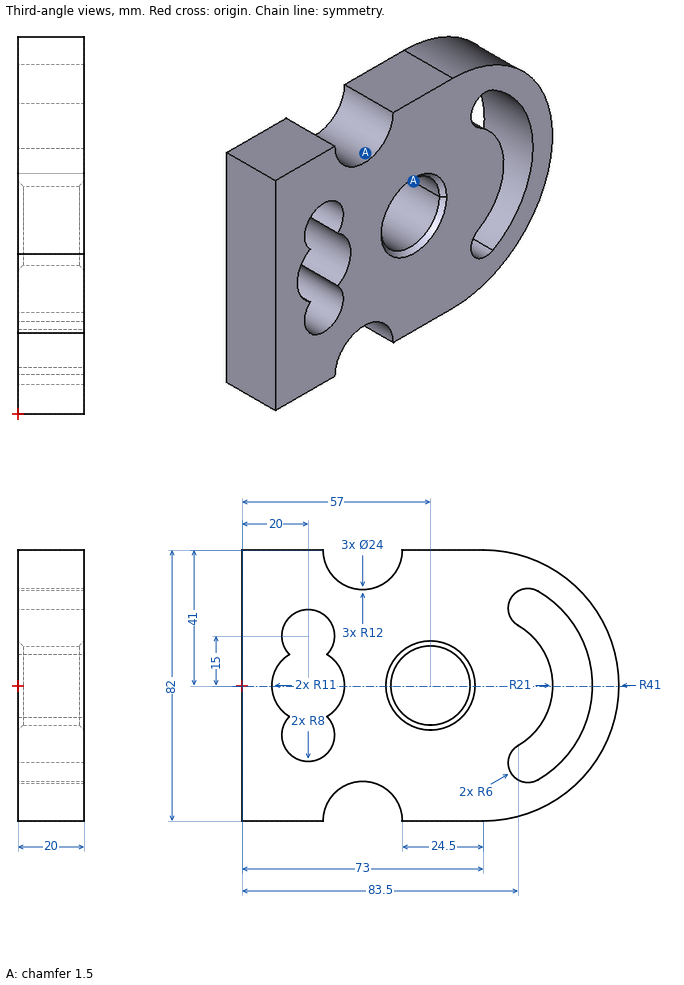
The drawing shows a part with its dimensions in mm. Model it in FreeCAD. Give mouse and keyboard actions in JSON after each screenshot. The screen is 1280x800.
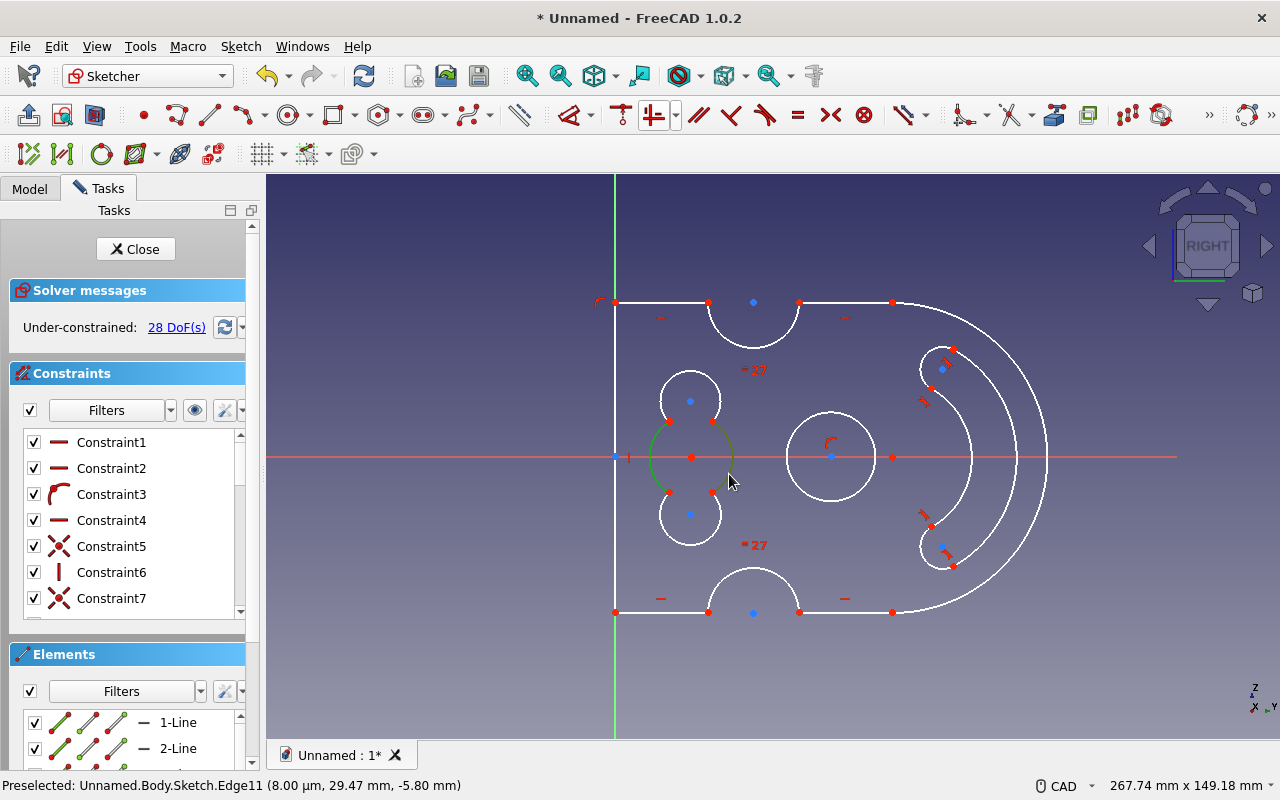
{"action": "key", "text": "e"}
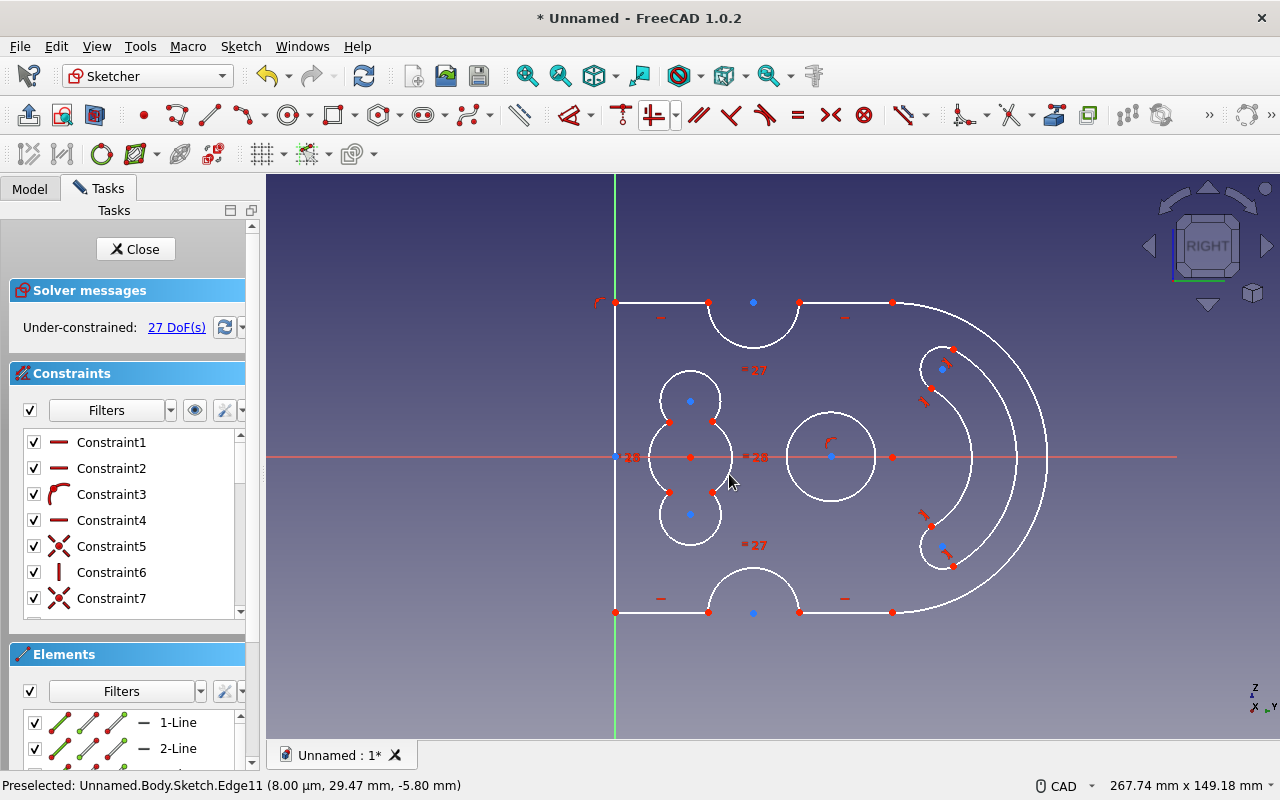
{"action": "left_click", "coordinate": [715, 383]}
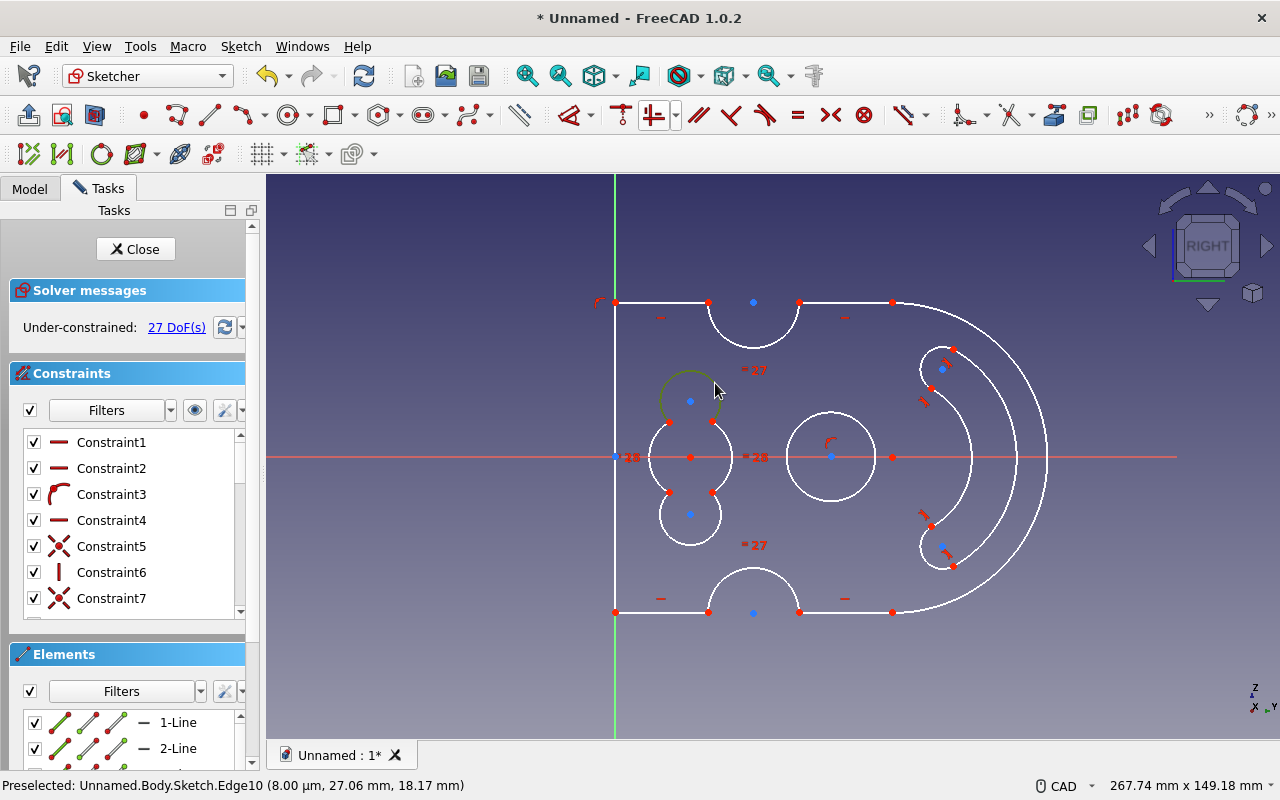
{"action": "left_click", "coordinate": [666, 532]}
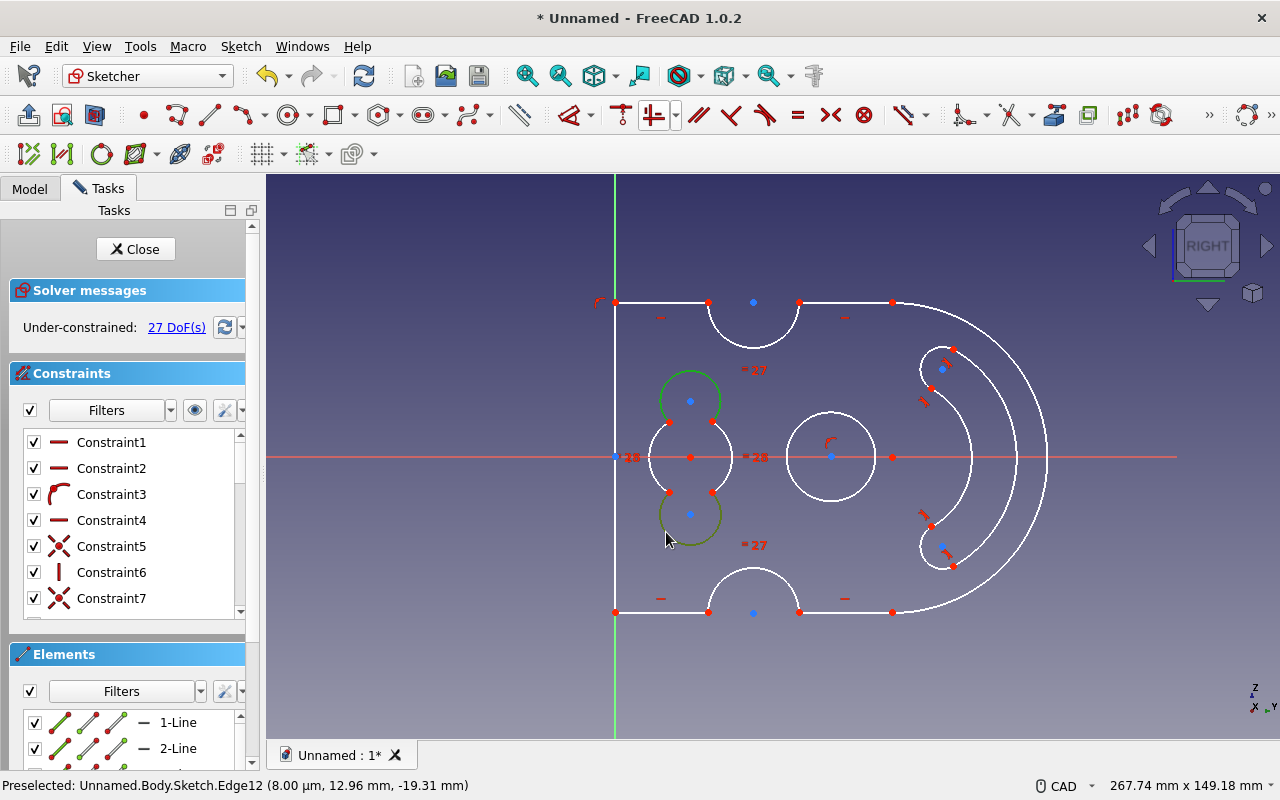
{"action": "left_click", "coordinate": [798, 116]}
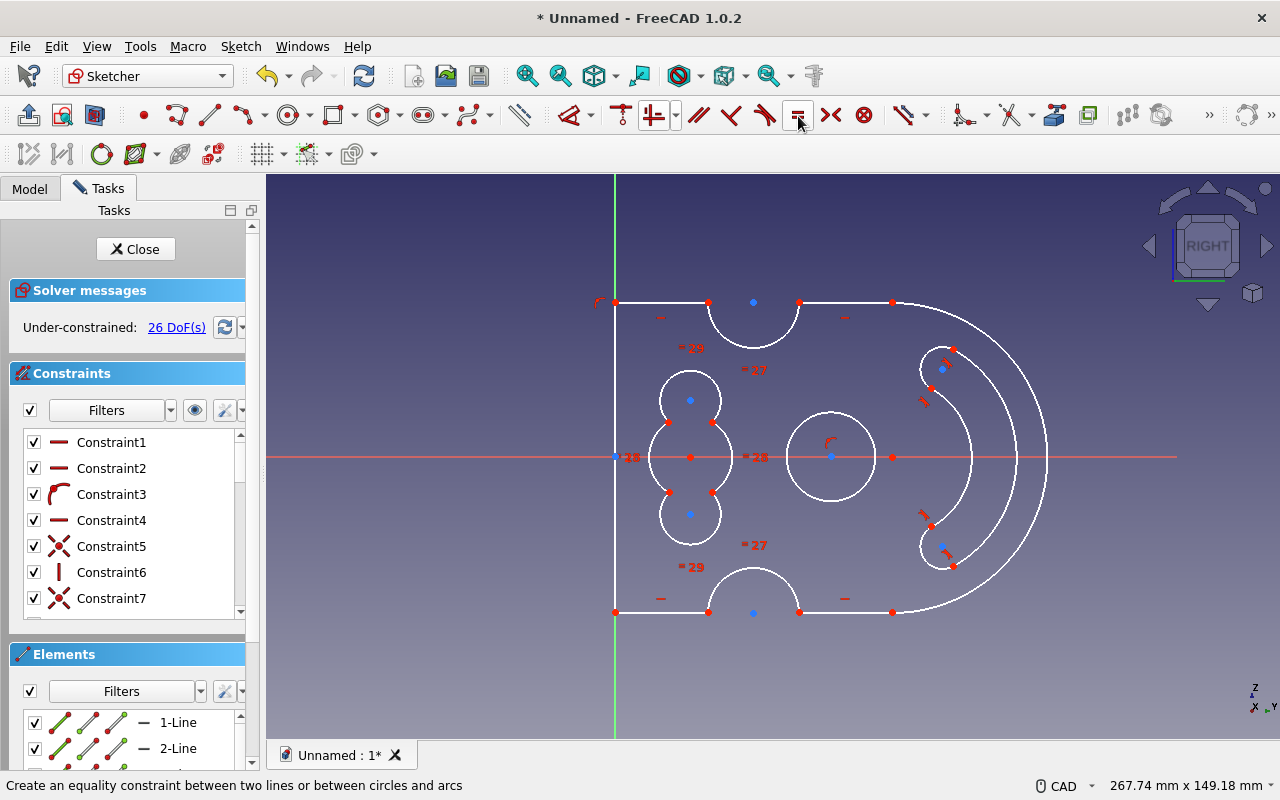
{"action": "left_click", "coordinate": [892, 458]}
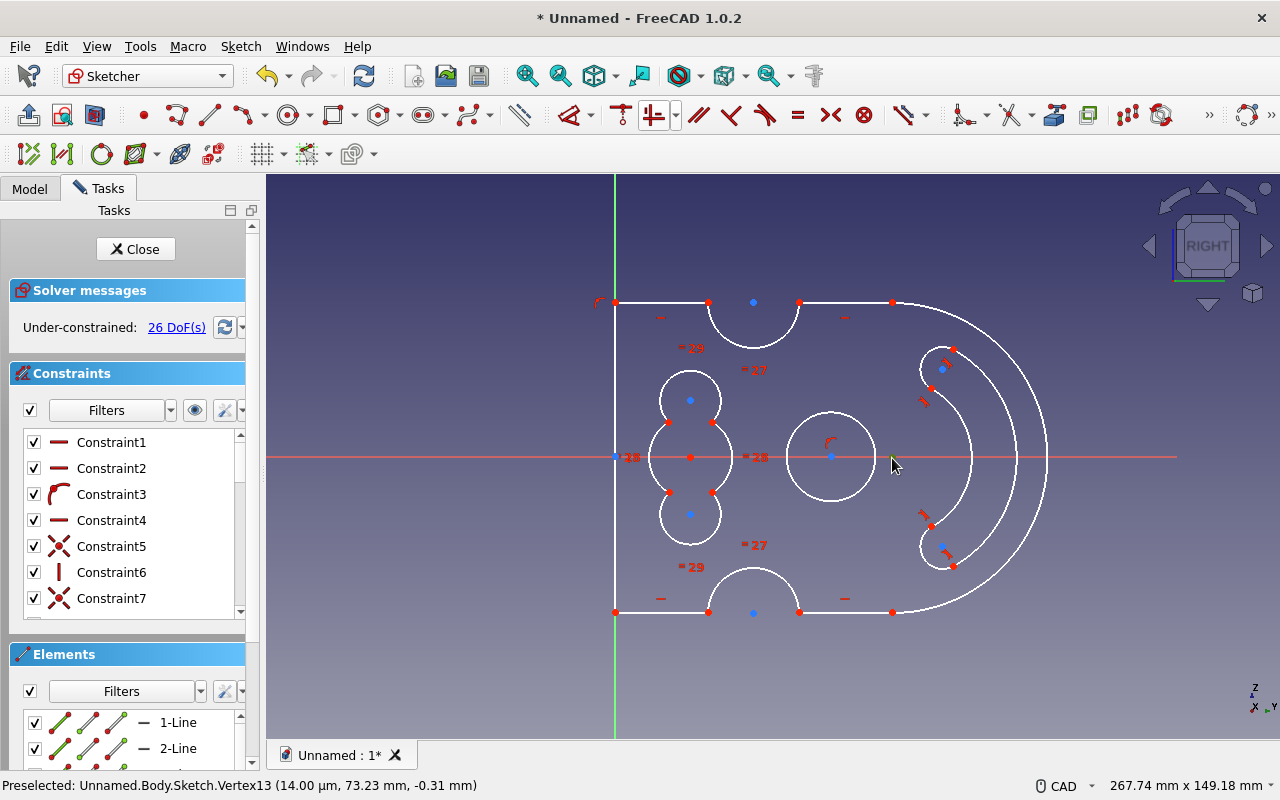
{"action": "left_click", "coordinate": [353, 457]}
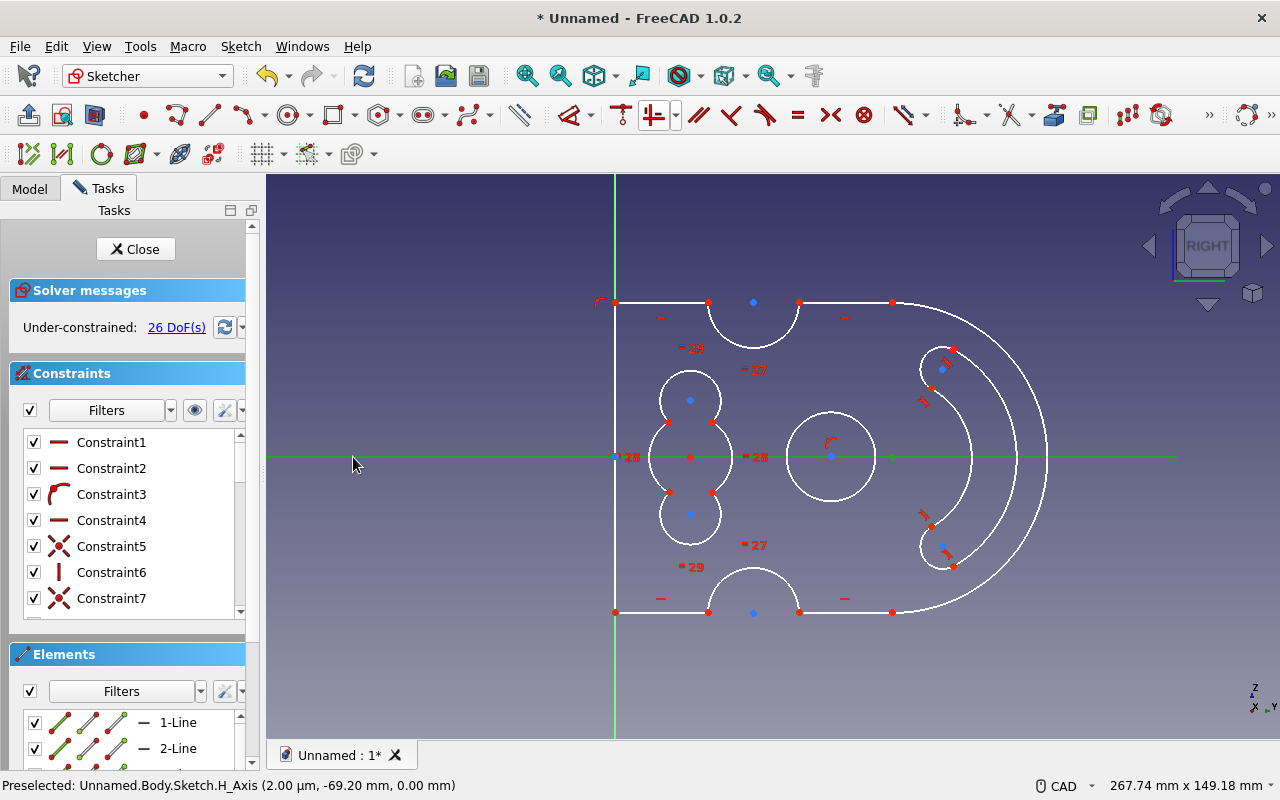
{"action": "left_click", "coordinate": [621, 116]}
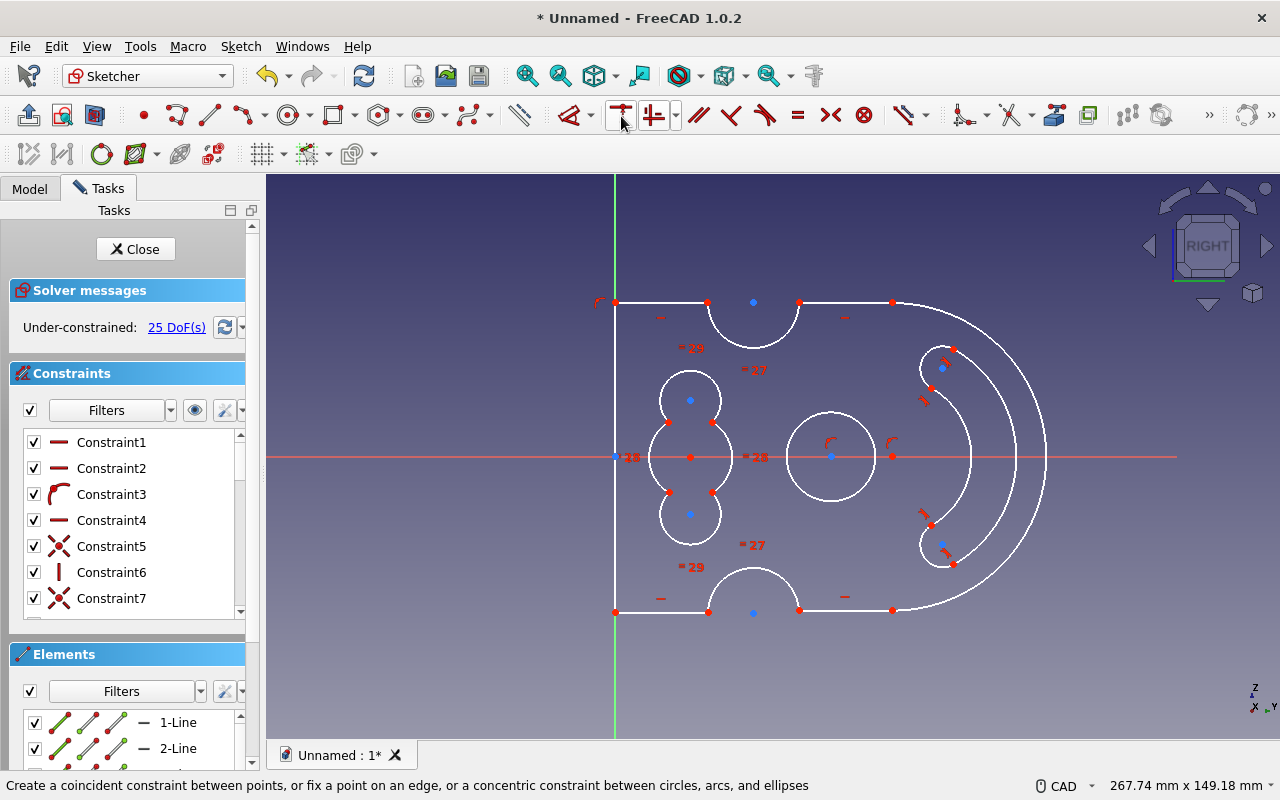
{"action": "left_click", "coordinate": [691, 457]}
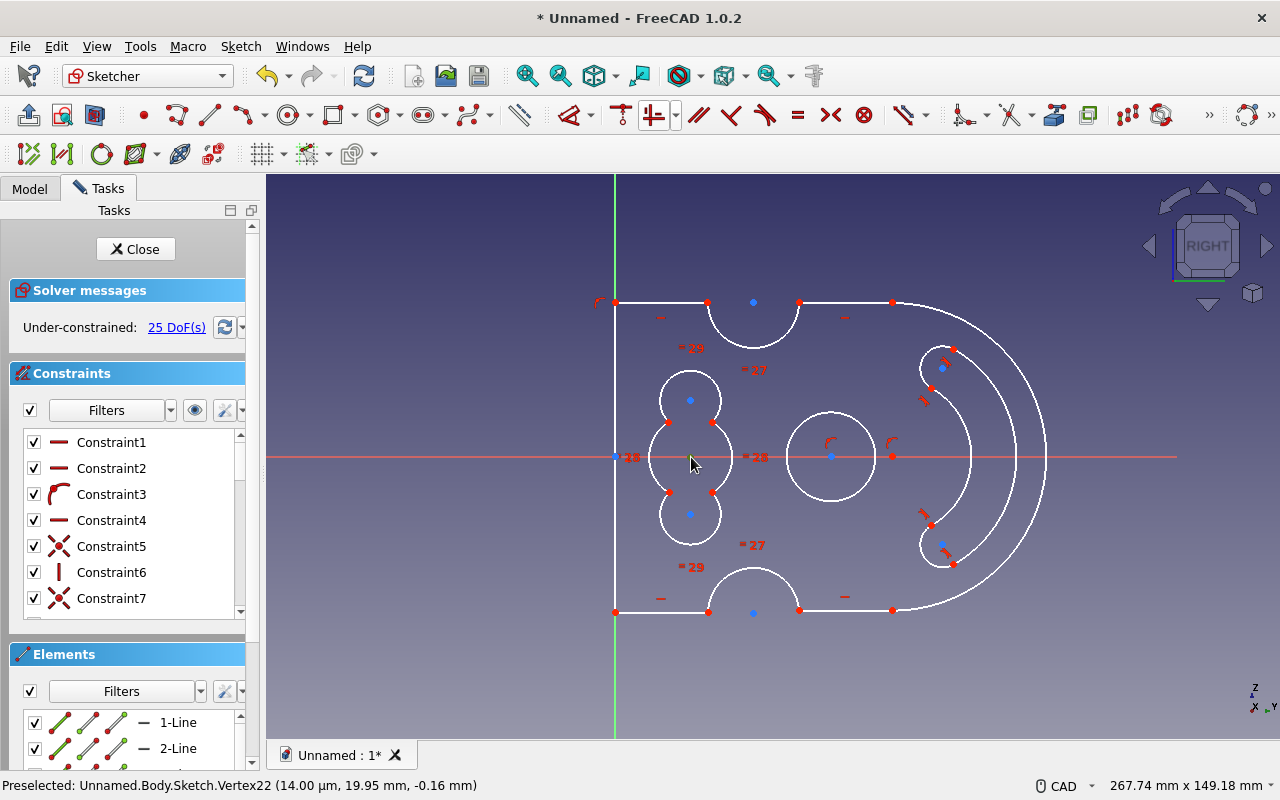
{"action": "left_click", "coordinate": [353, 457]}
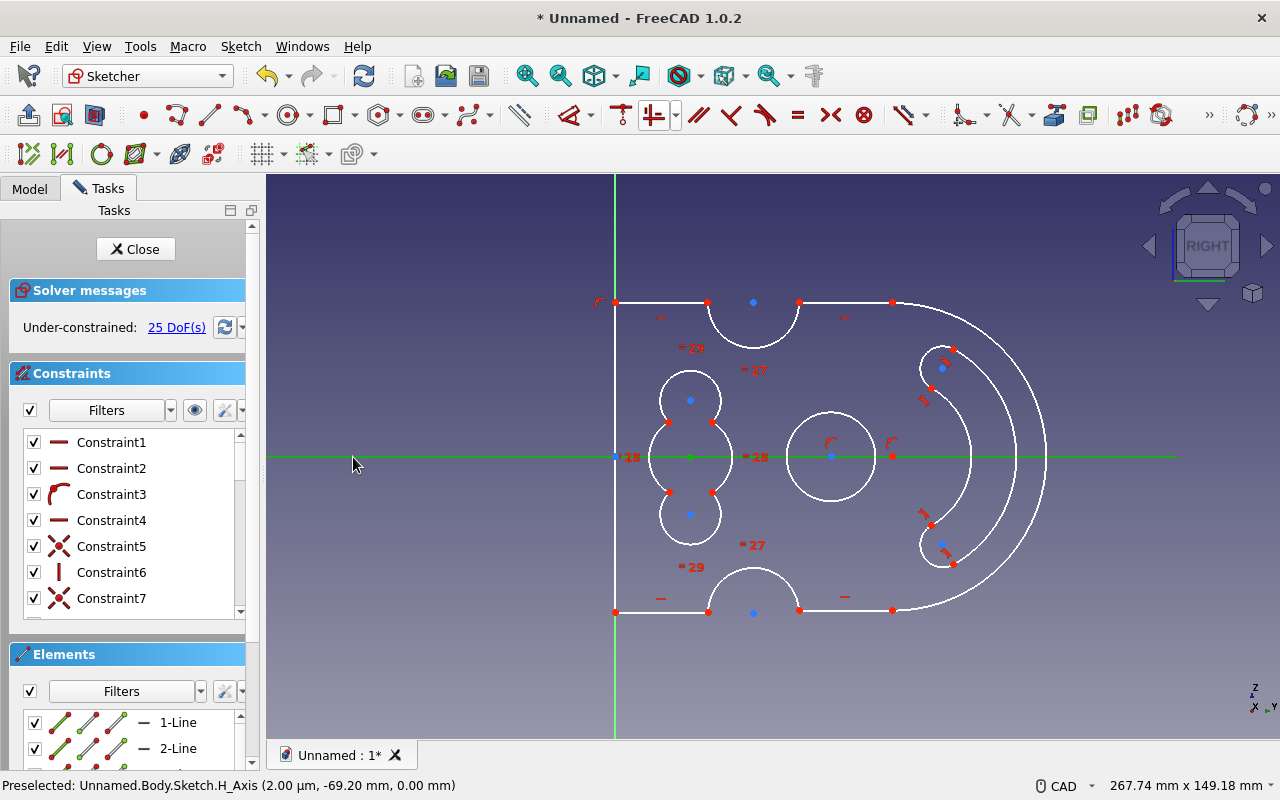
{"action": "key", "text": "c"}